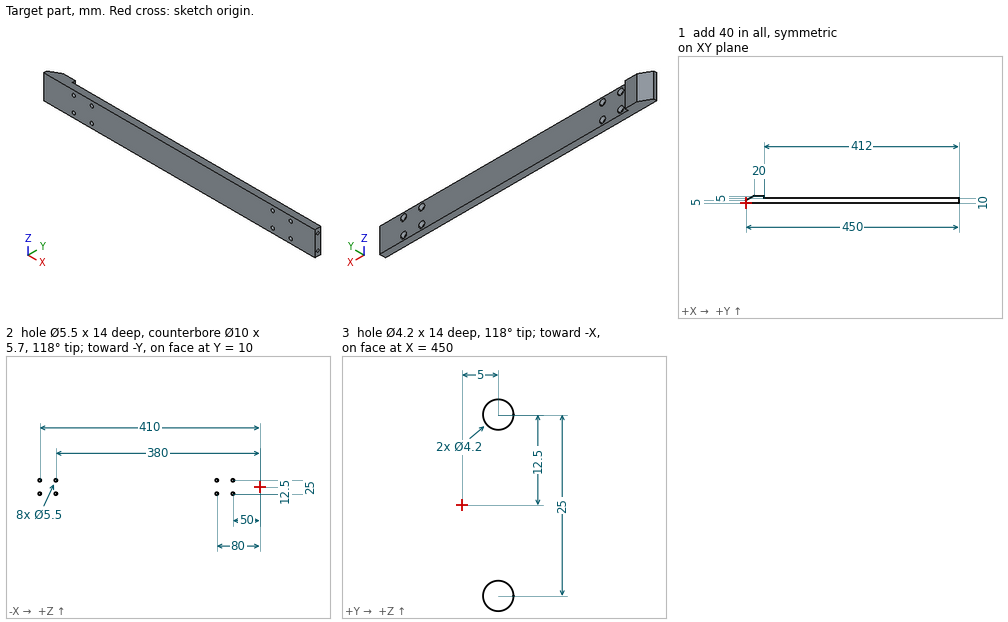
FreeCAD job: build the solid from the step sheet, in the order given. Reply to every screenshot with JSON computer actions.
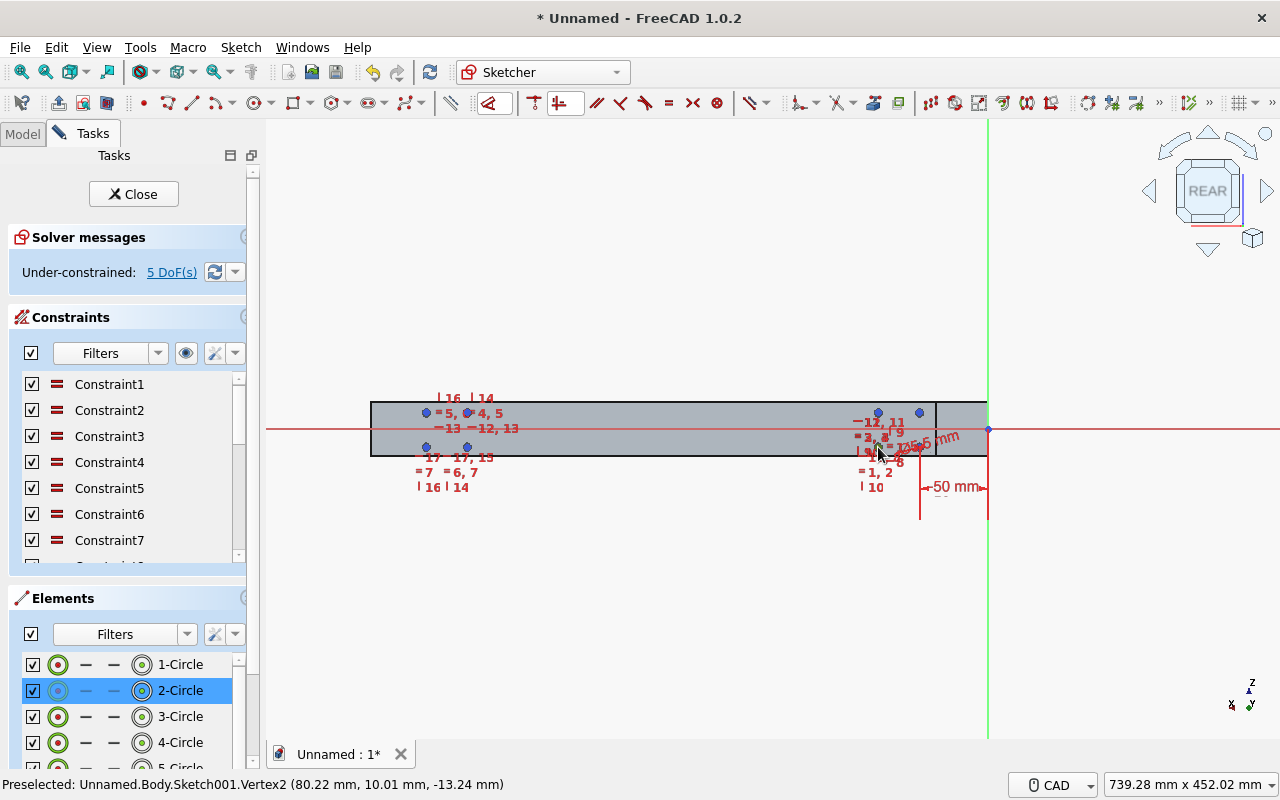
{"action": "key", "text": "l"}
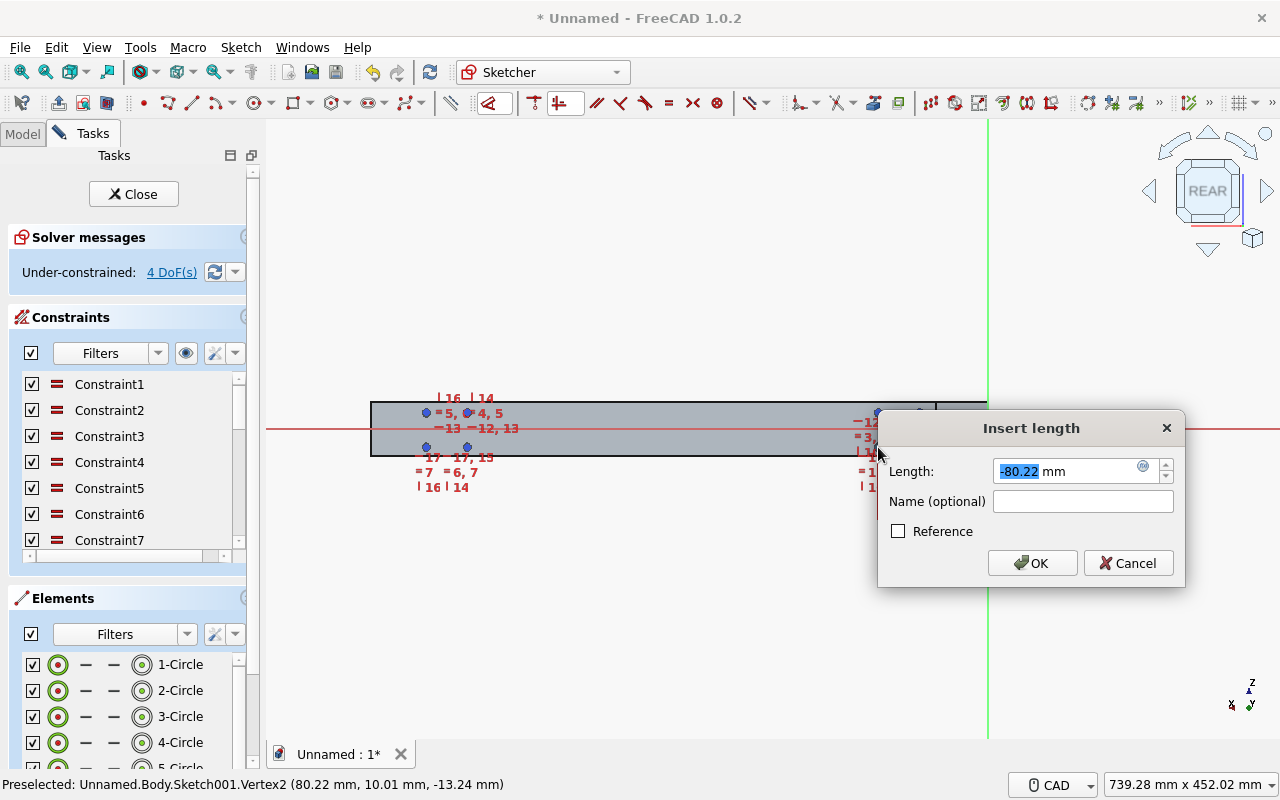
{"action": "type", "text": "-80"}
{"action": "key", "text": "Return"}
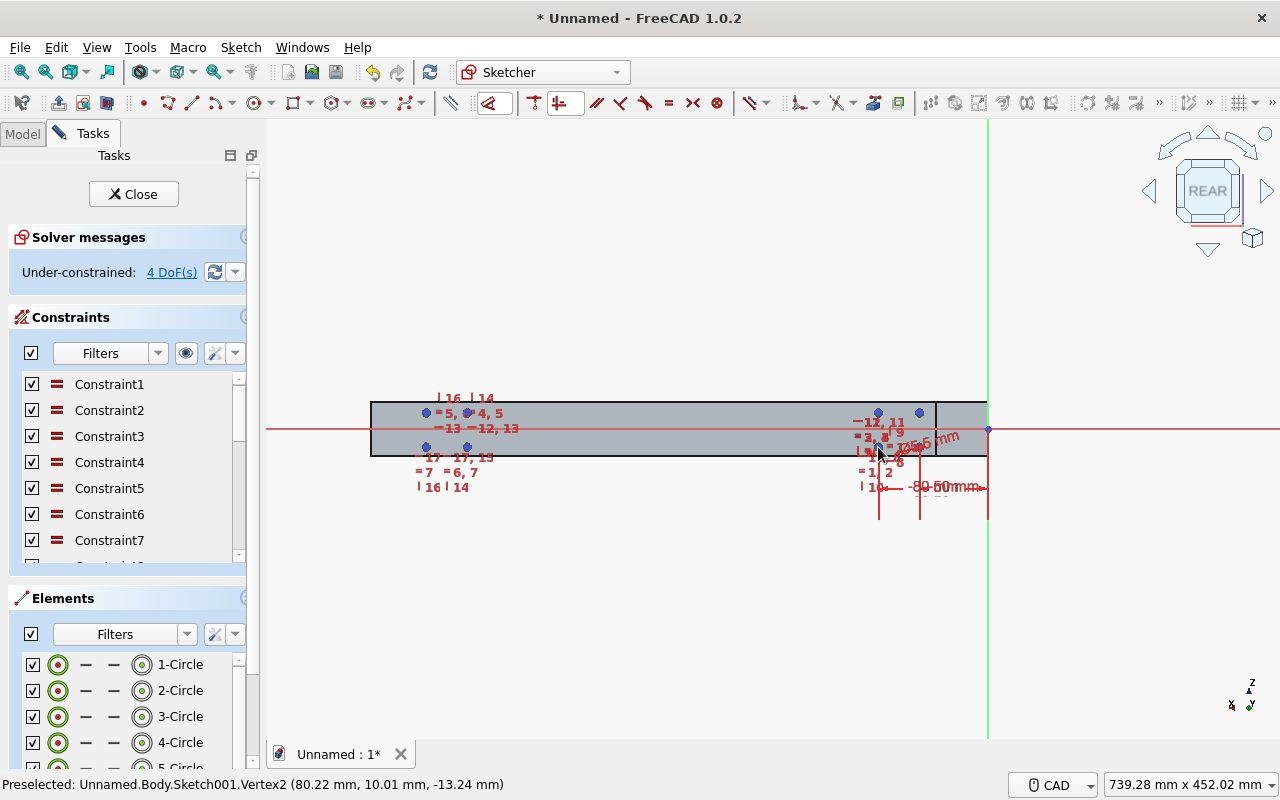
{"action": "left_click", "coordinate": [467, 413]}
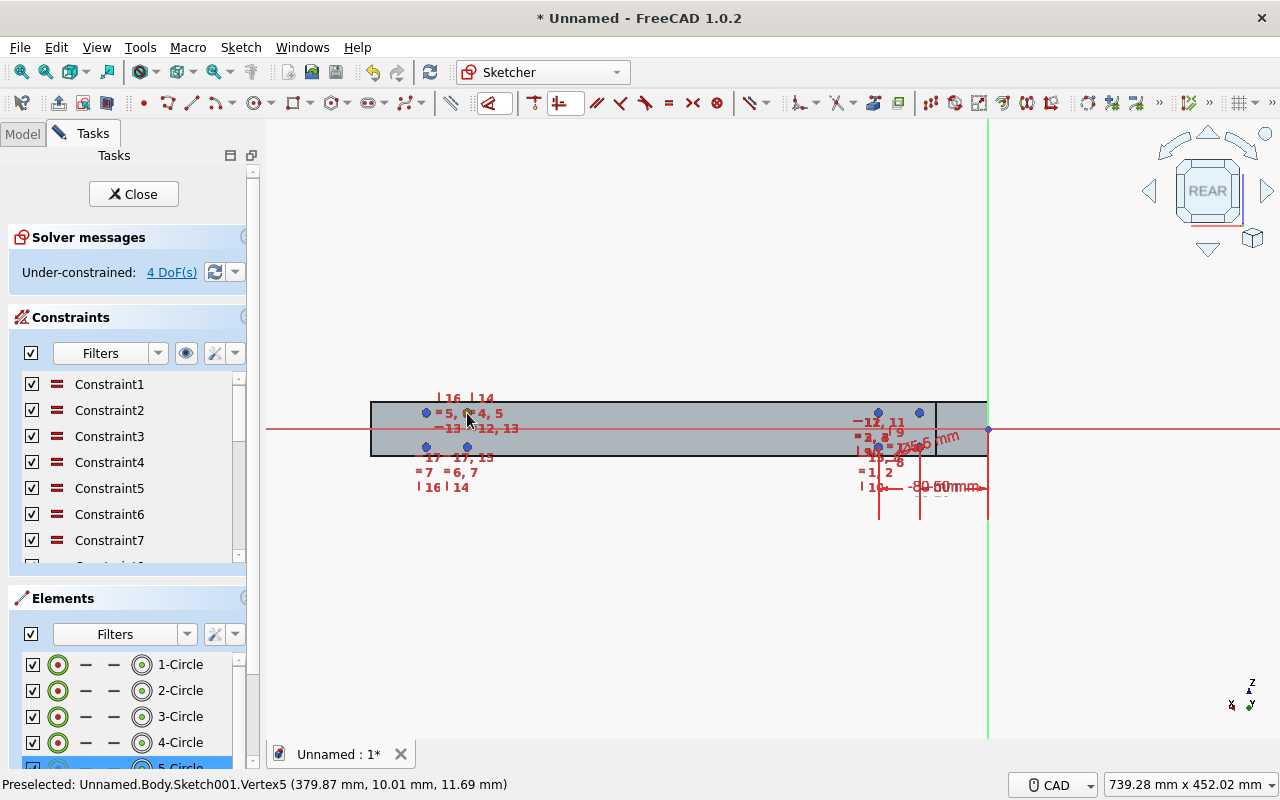
{"action": "left_click", "coordinate": [506, 104]}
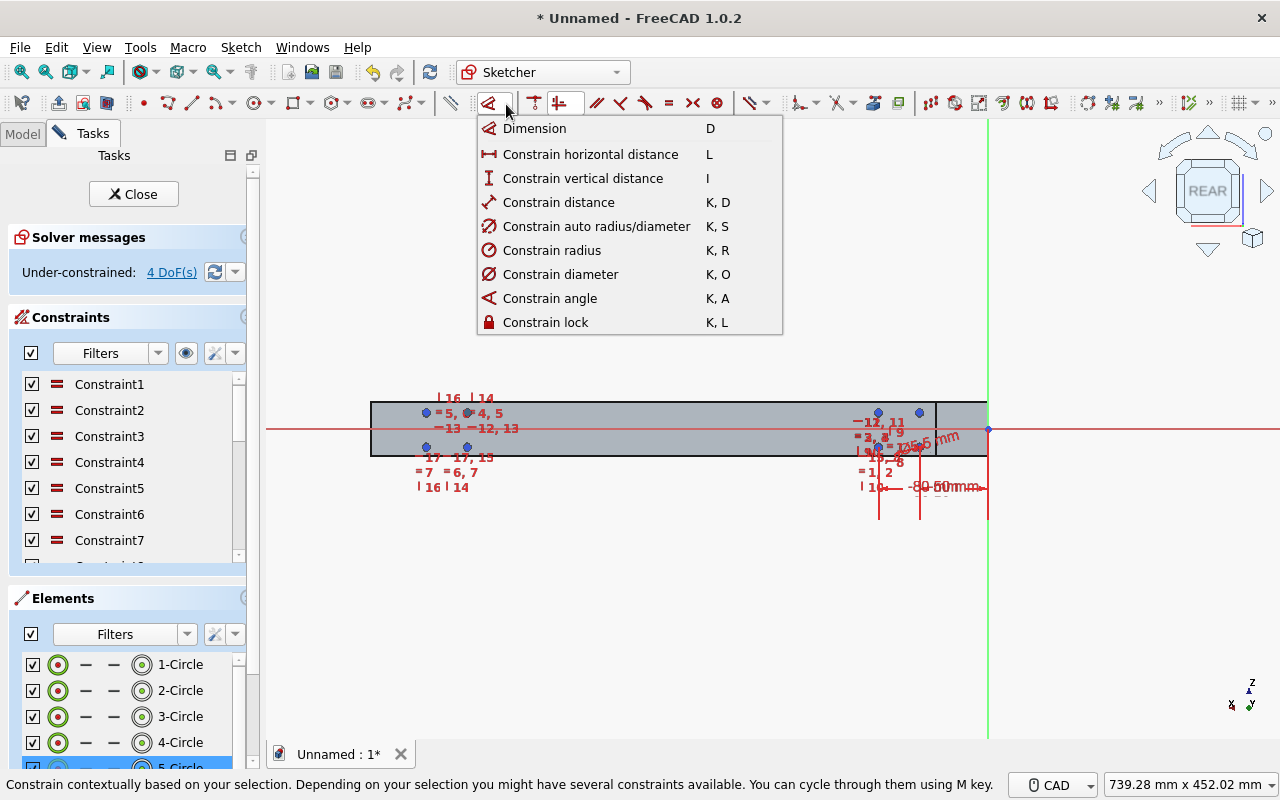
{"action": "left_click", "coordinate": [630, 154]}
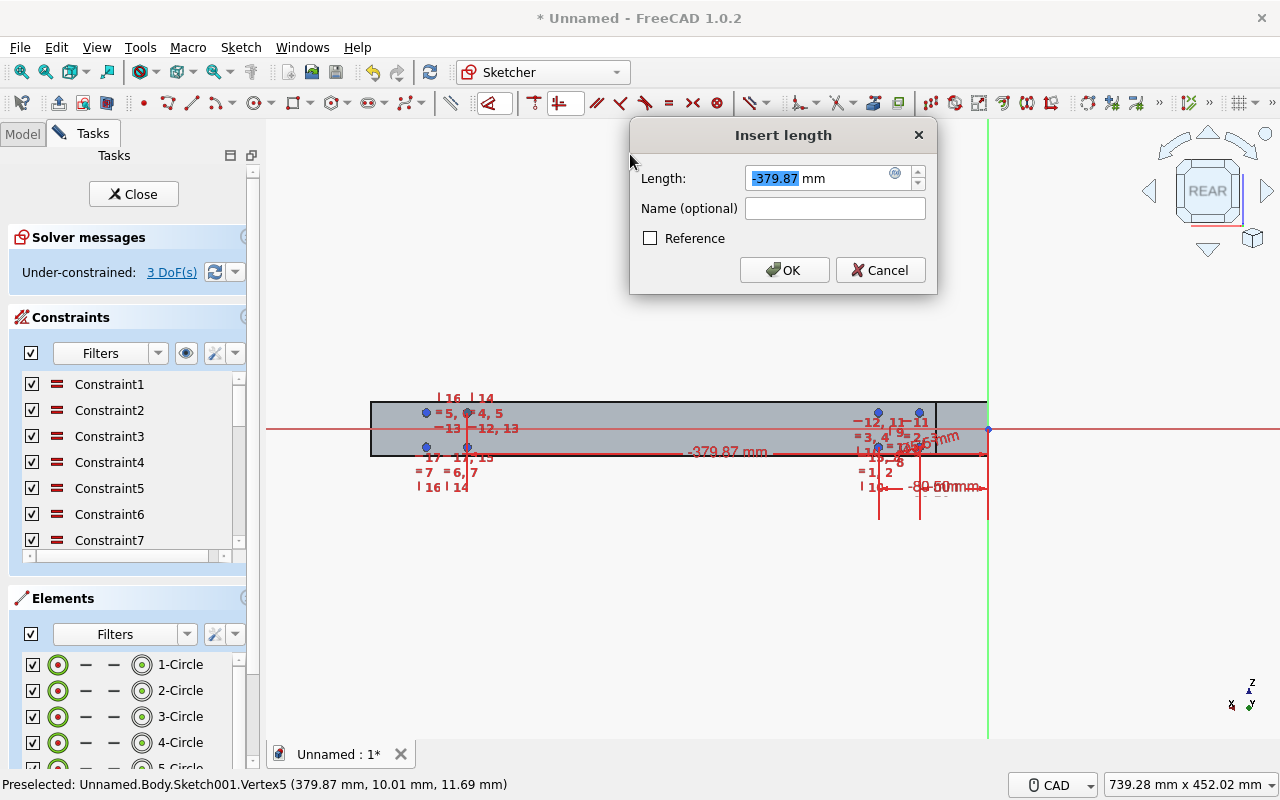
{"action": "type", "text": "-380"}
{"action": "key", "text": "Return"}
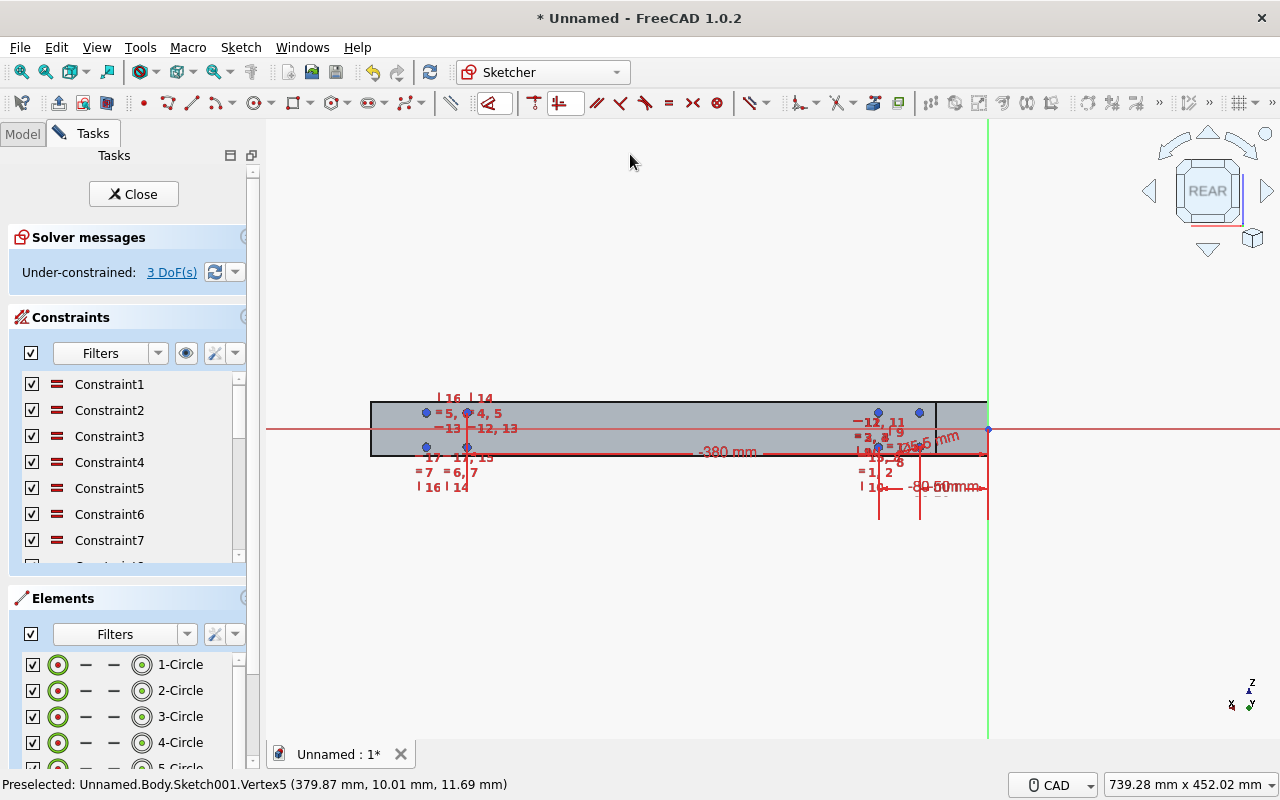
{"action": "left_click", "coordinate": [426, 413]}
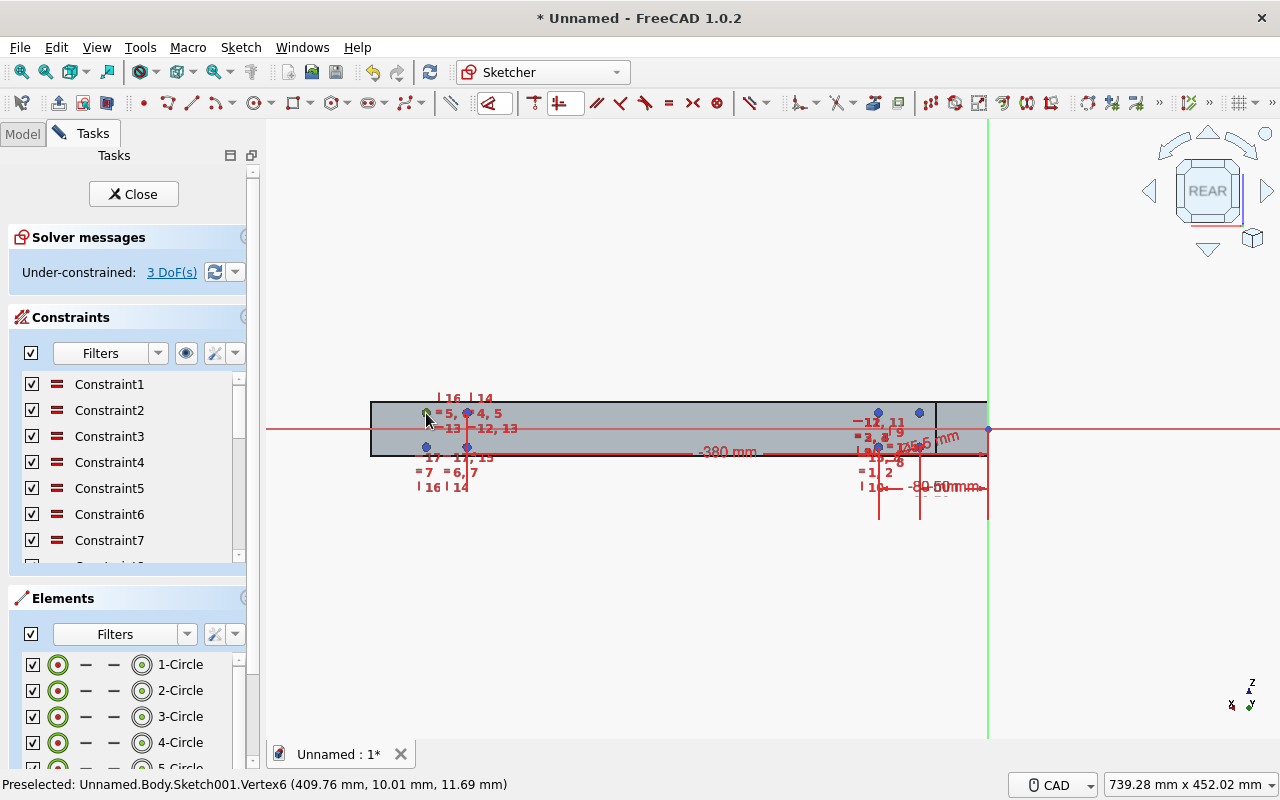
{"action": "key", "text": "l"}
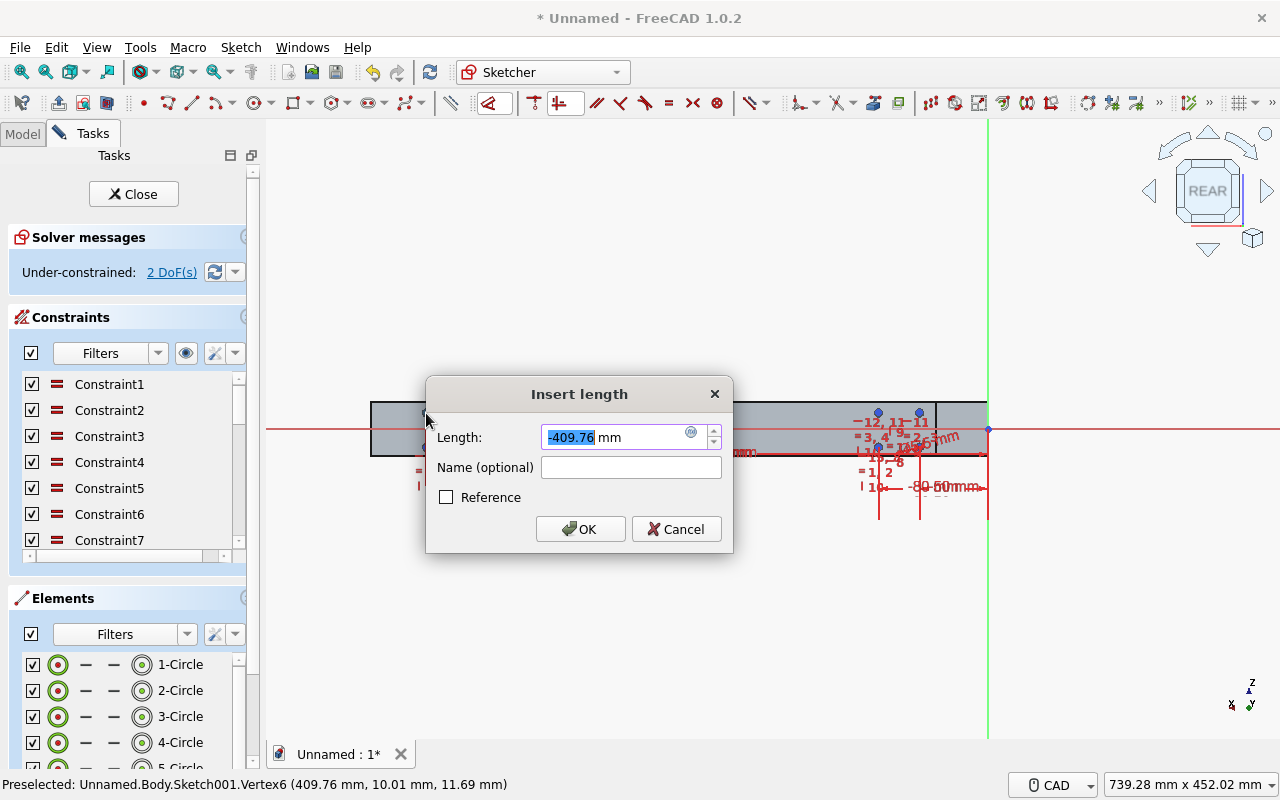
{"action": "type", "text": "-410"}
{"action": "key", "text": "Return"}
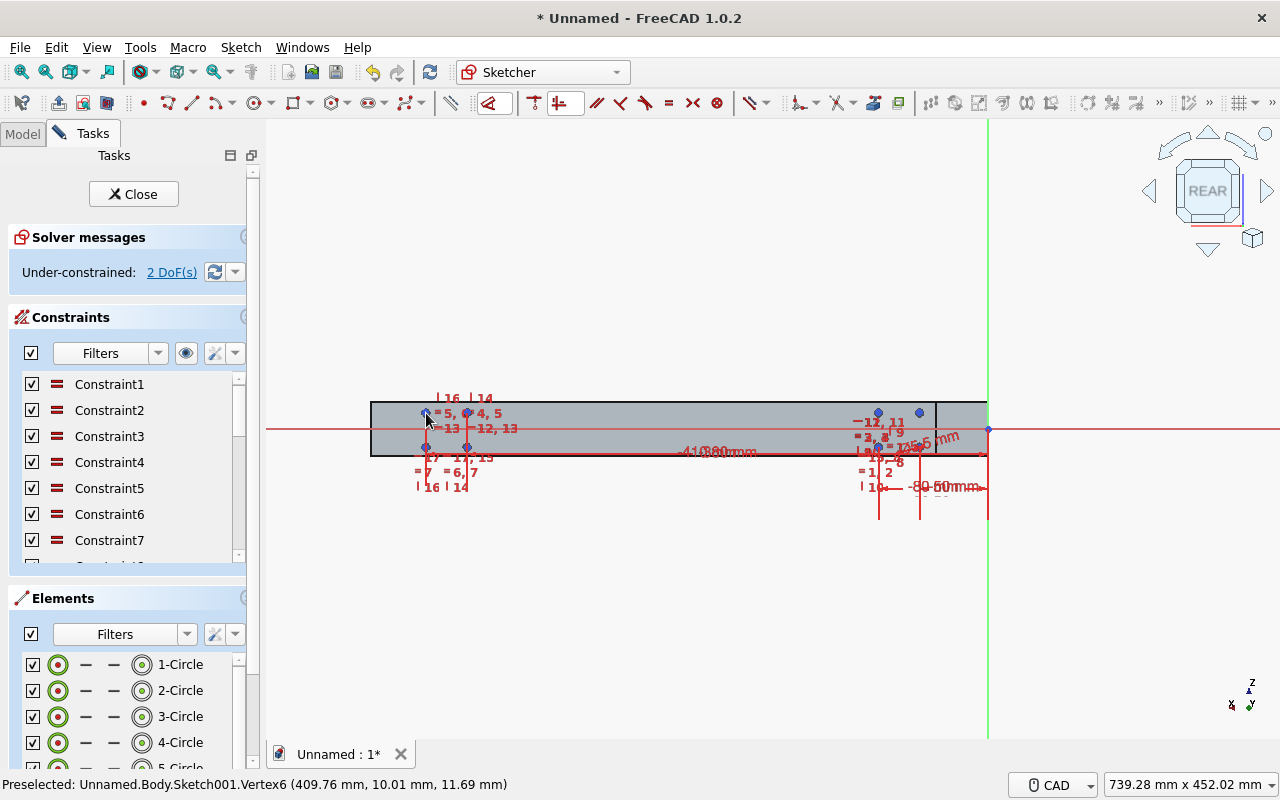
{"action": "left_click", "coordinate": [920, 447]}